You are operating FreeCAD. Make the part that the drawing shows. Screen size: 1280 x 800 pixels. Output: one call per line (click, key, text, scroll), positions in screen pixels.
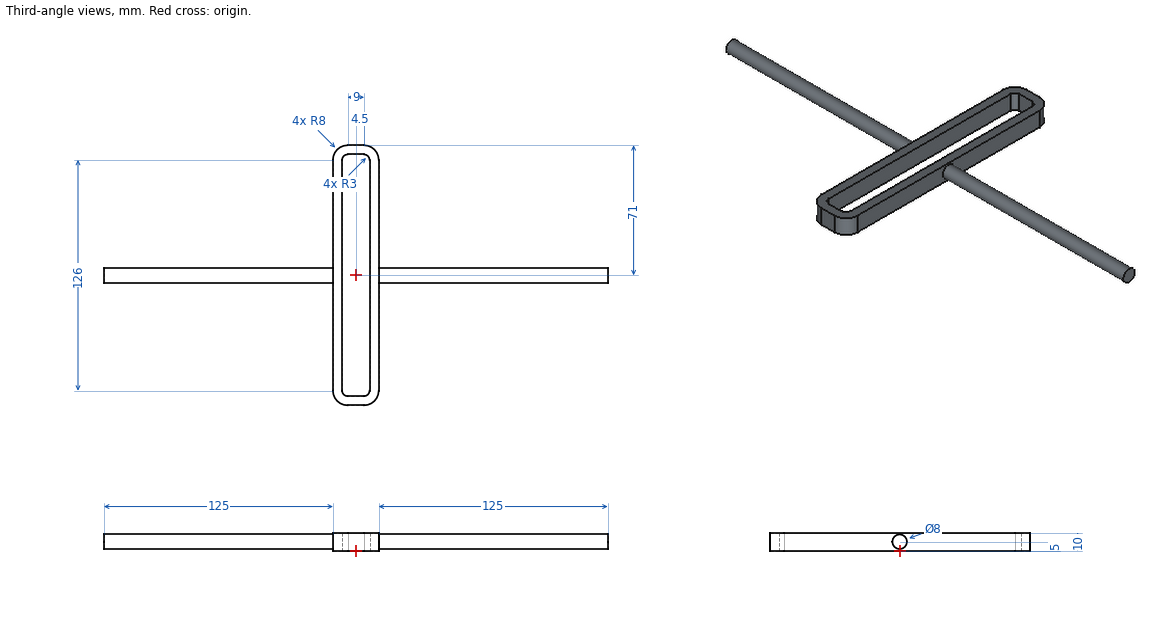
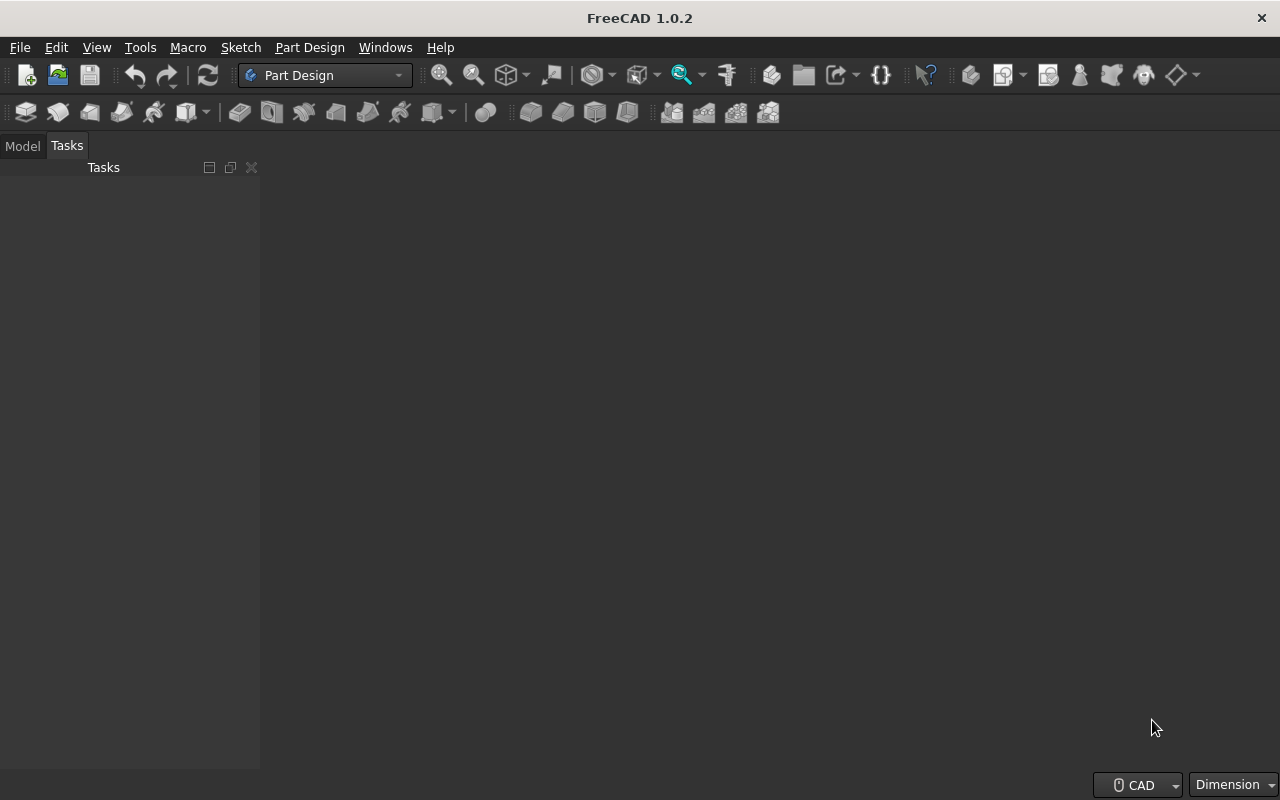
click(26, 76)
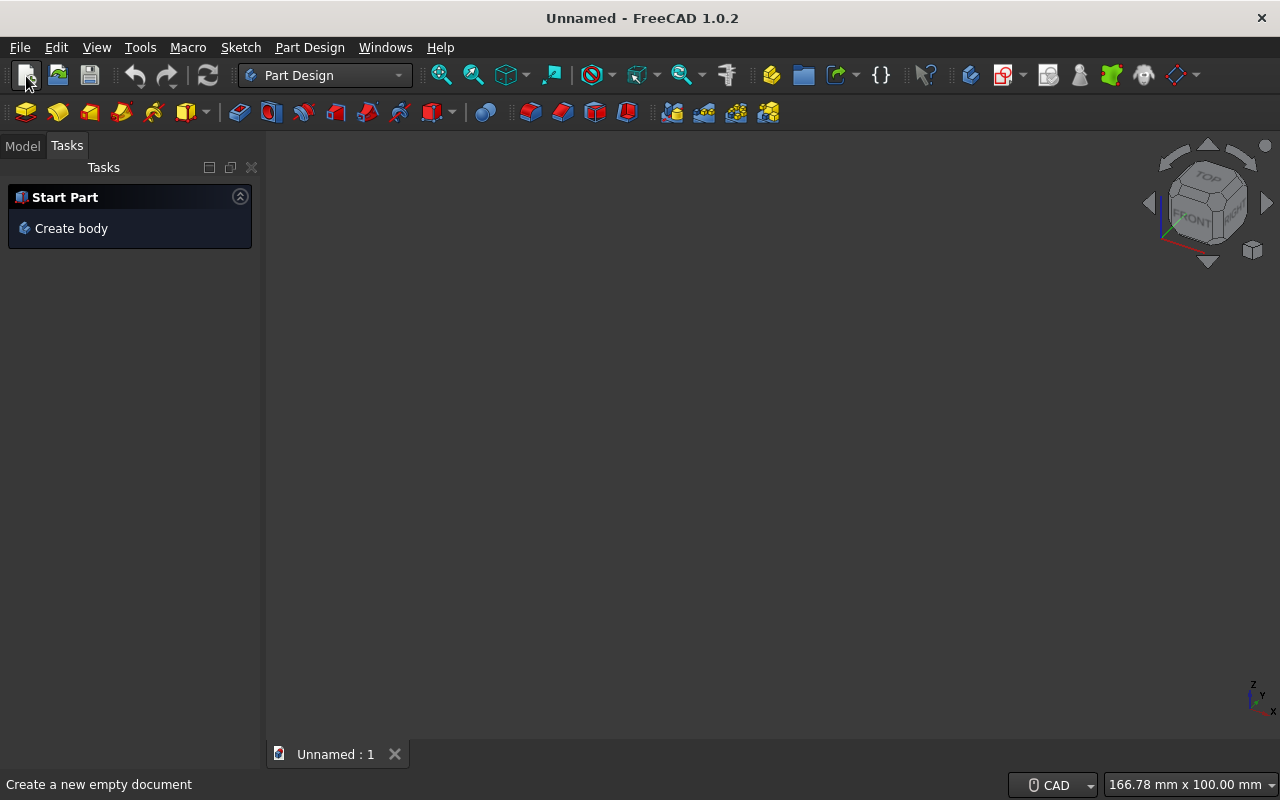
click(1004, 76)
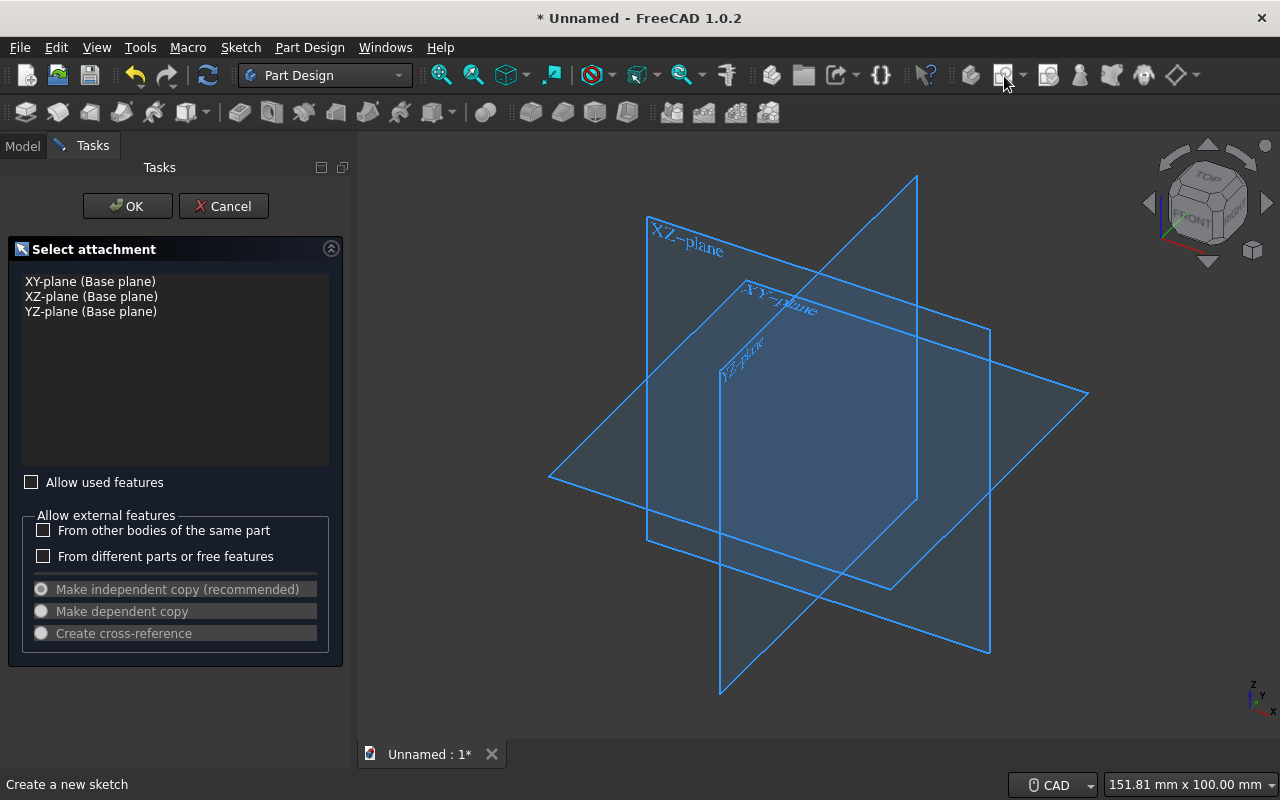
click(82, 282)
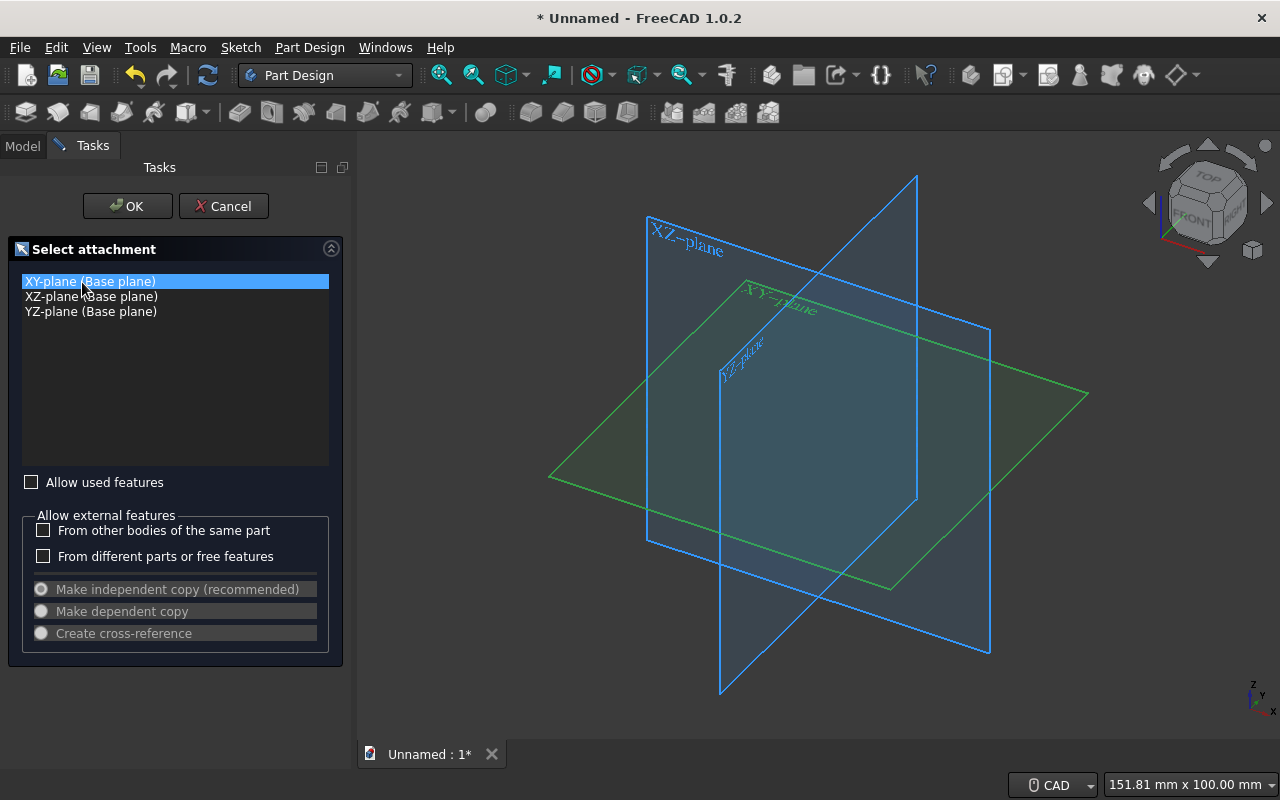
click(128, 206)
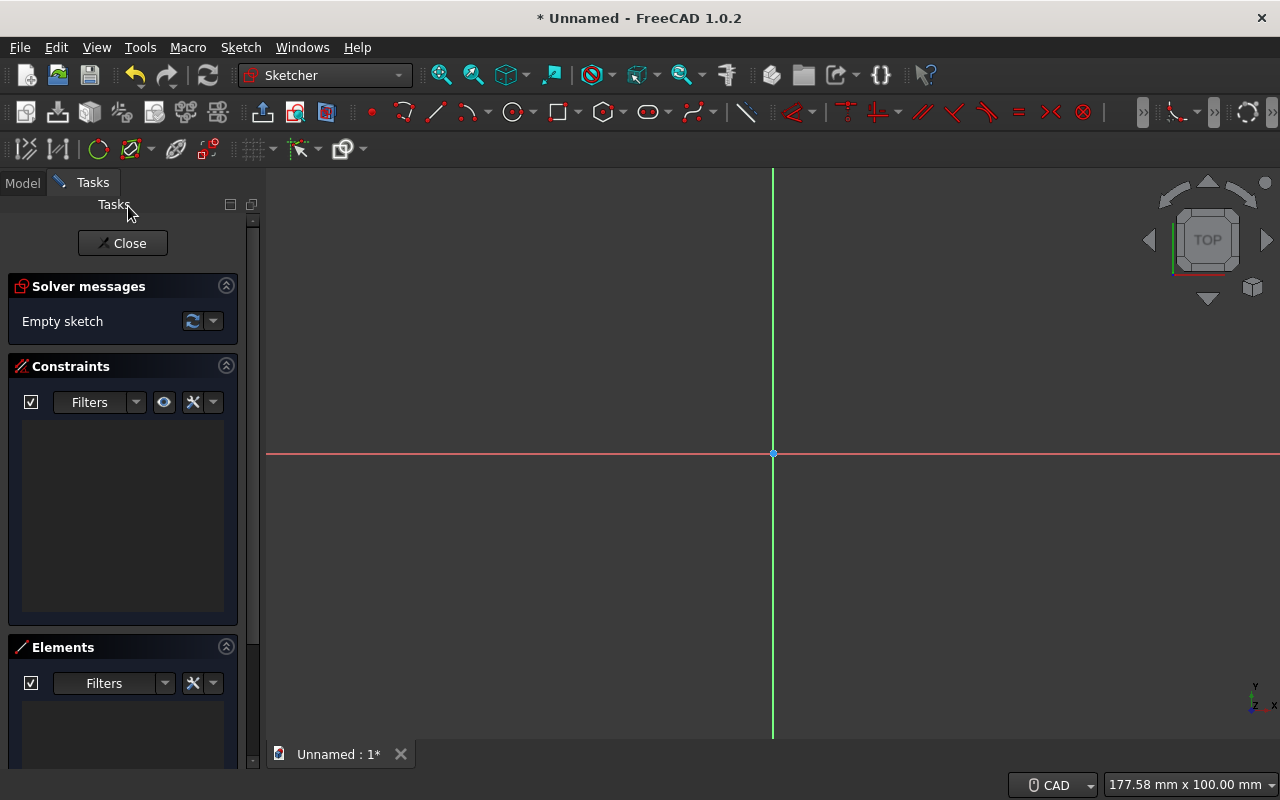
scroll(649, 454, down, 4)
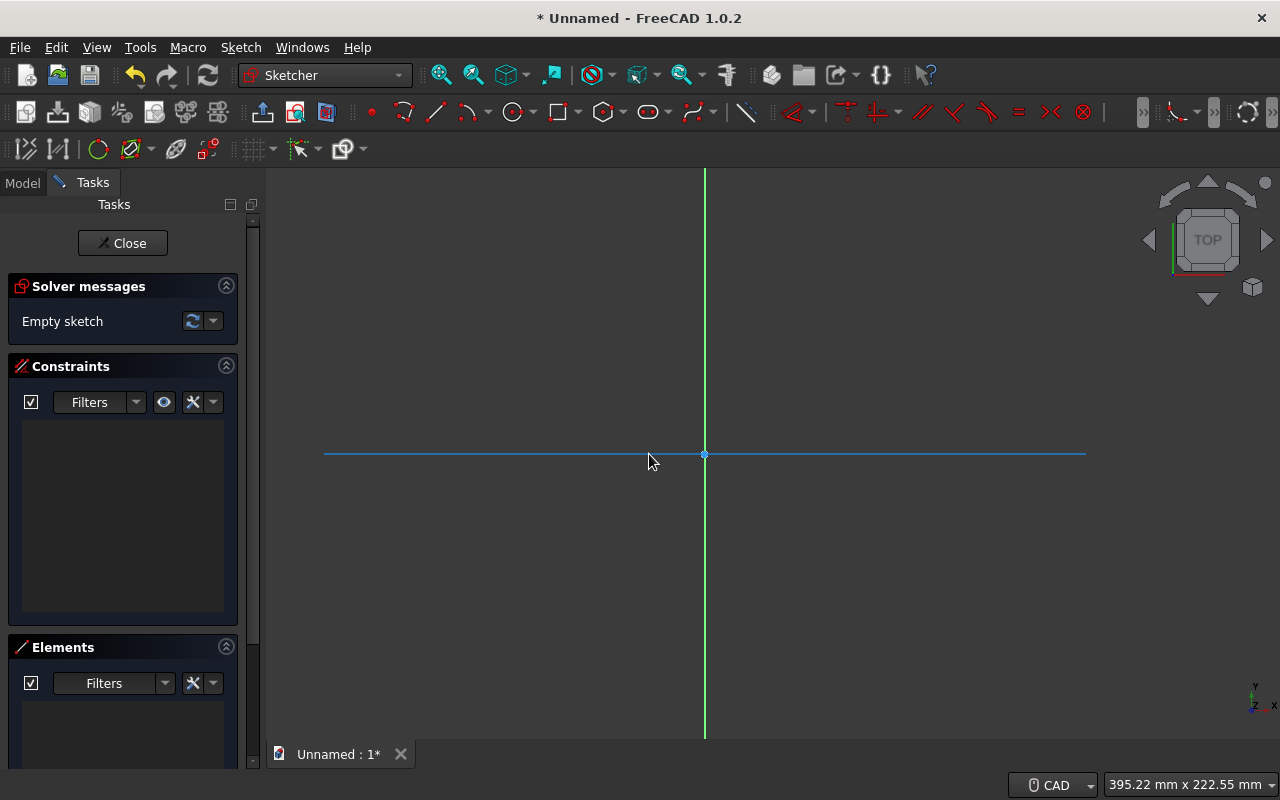
click(436, 112)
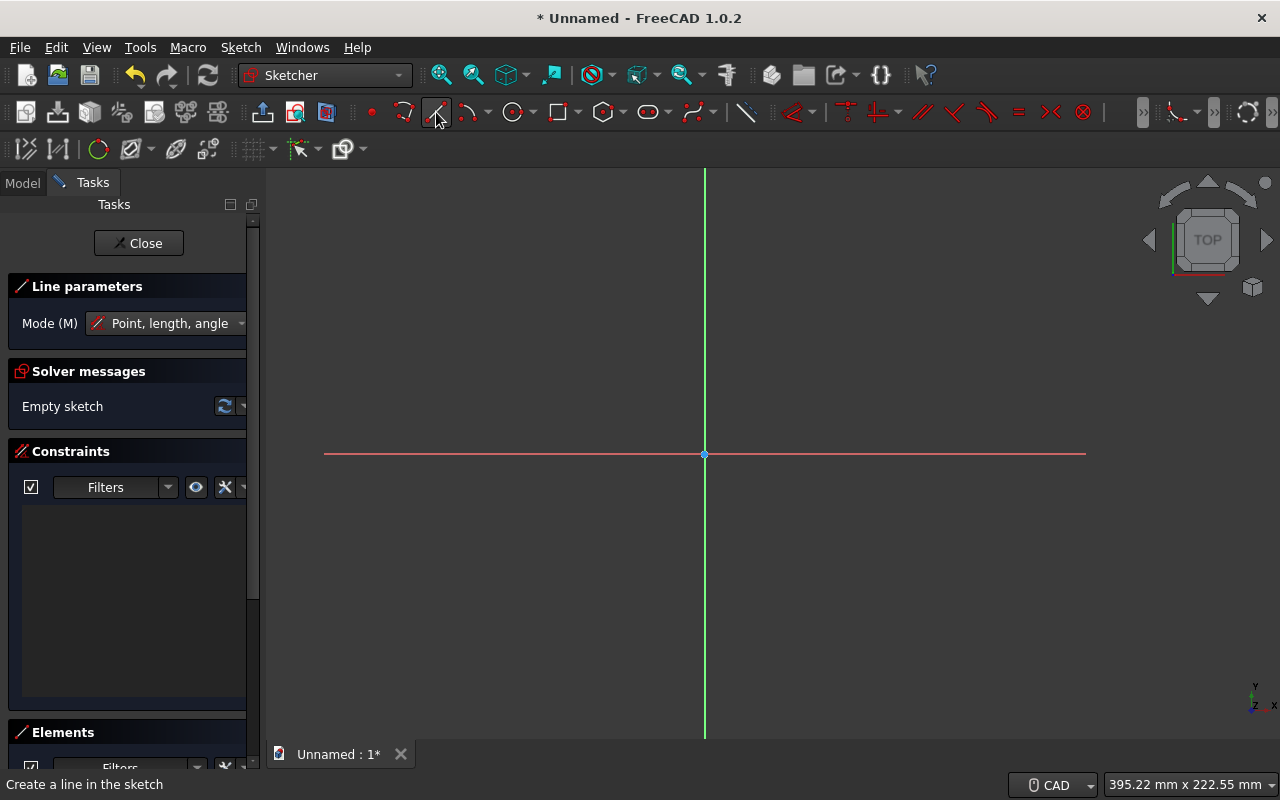
scroll(716, 272, up, 2)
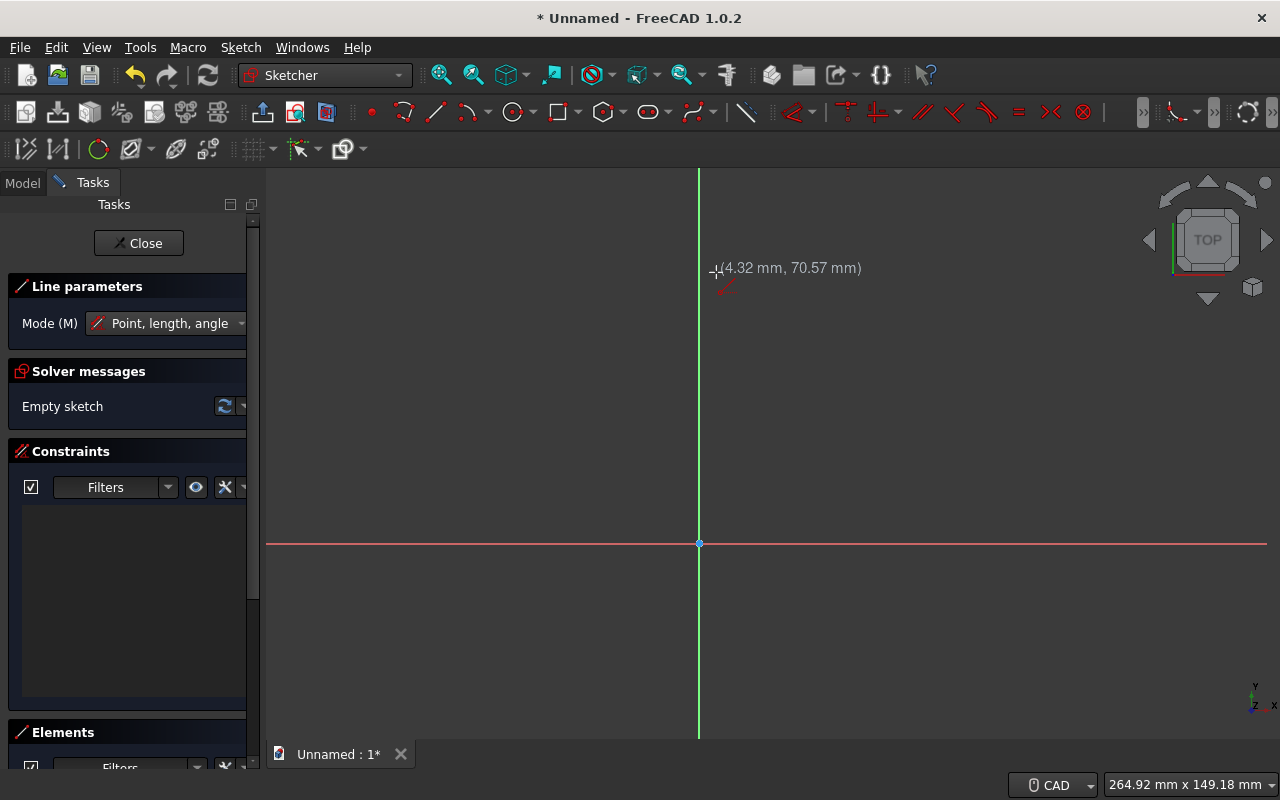
click(716, 272)
click(682, 272)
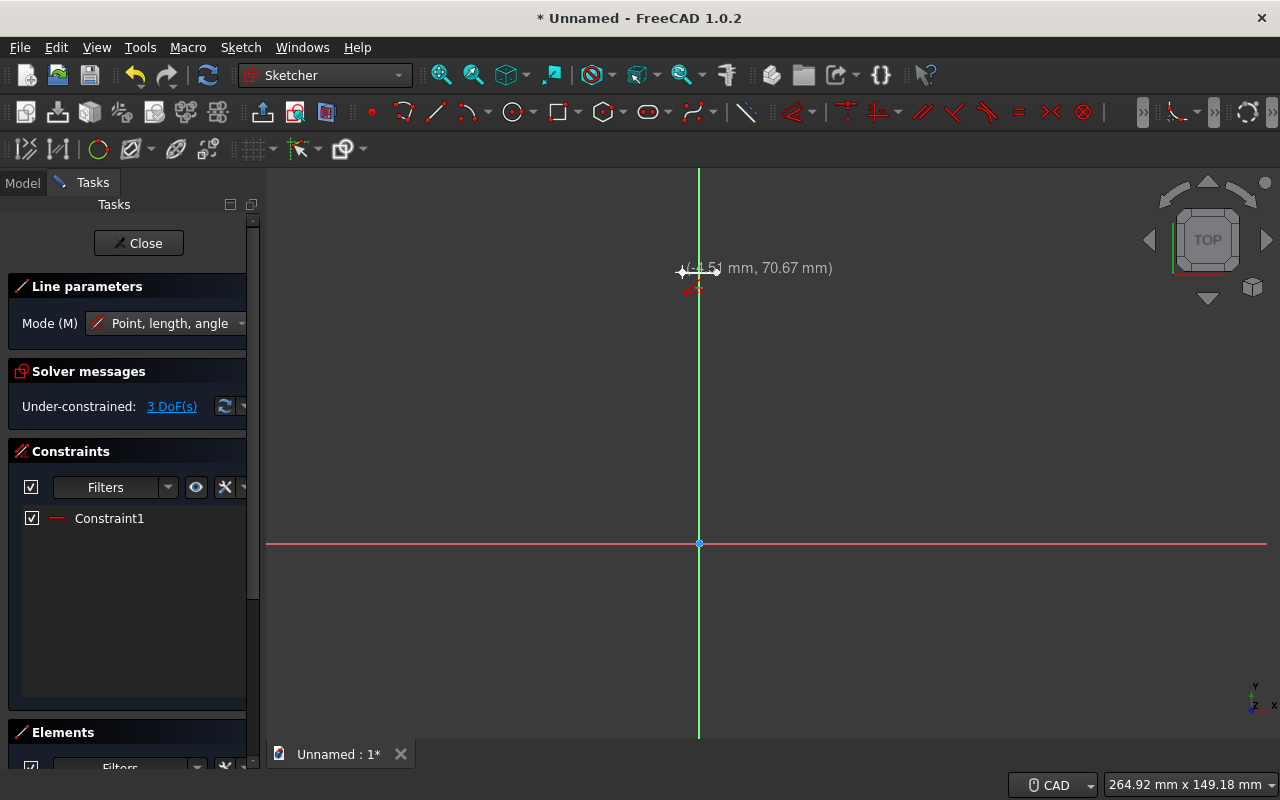
click(651, 302)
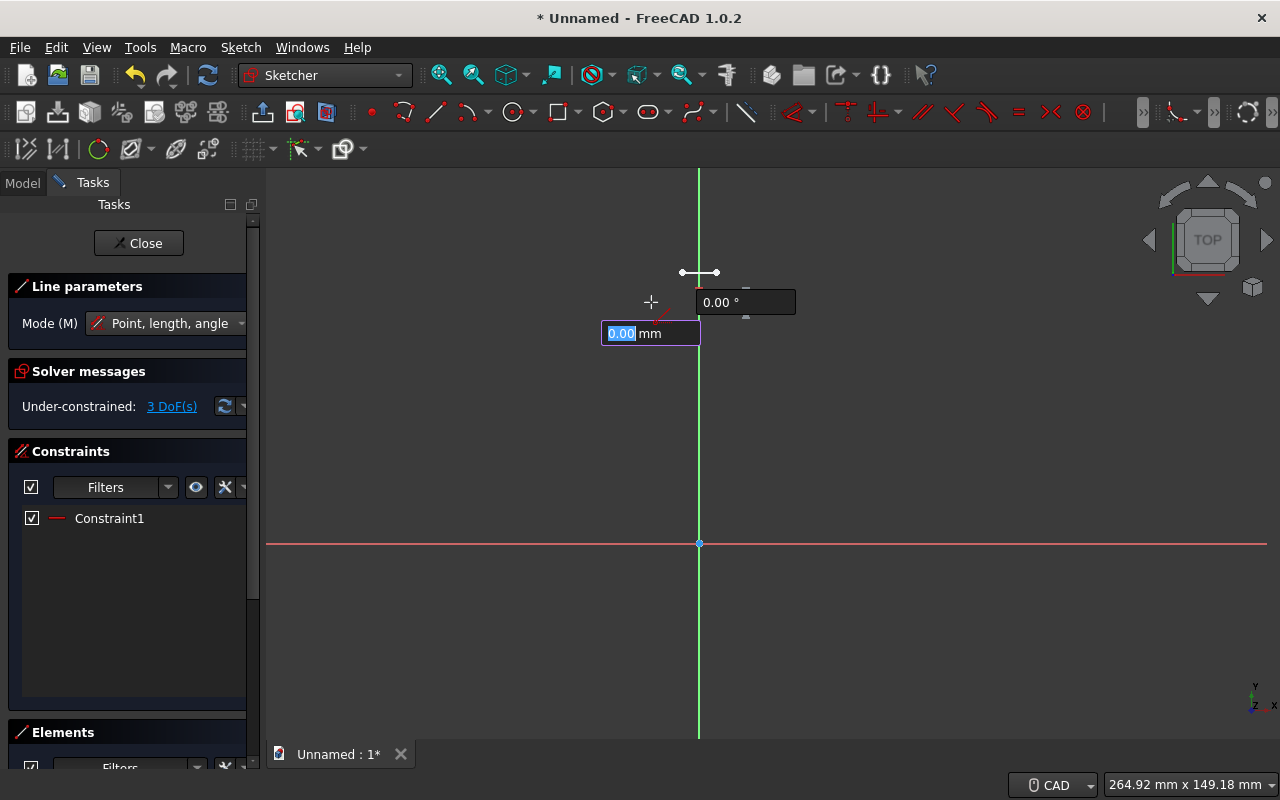
scroll(715, 271, down, 2)